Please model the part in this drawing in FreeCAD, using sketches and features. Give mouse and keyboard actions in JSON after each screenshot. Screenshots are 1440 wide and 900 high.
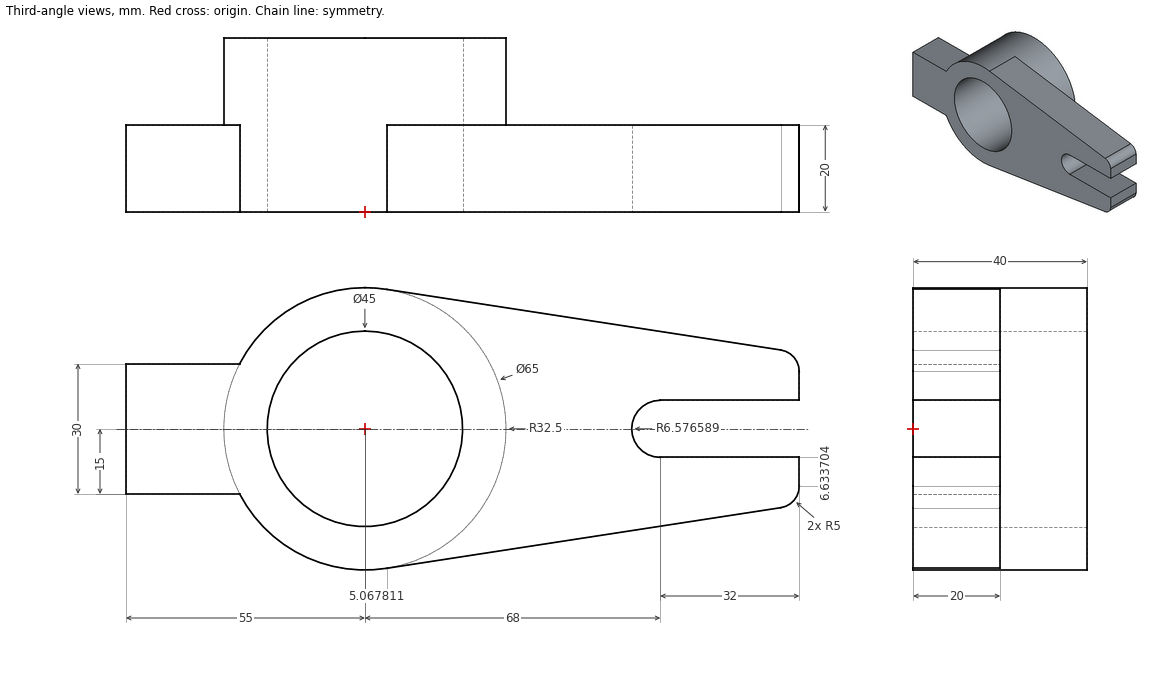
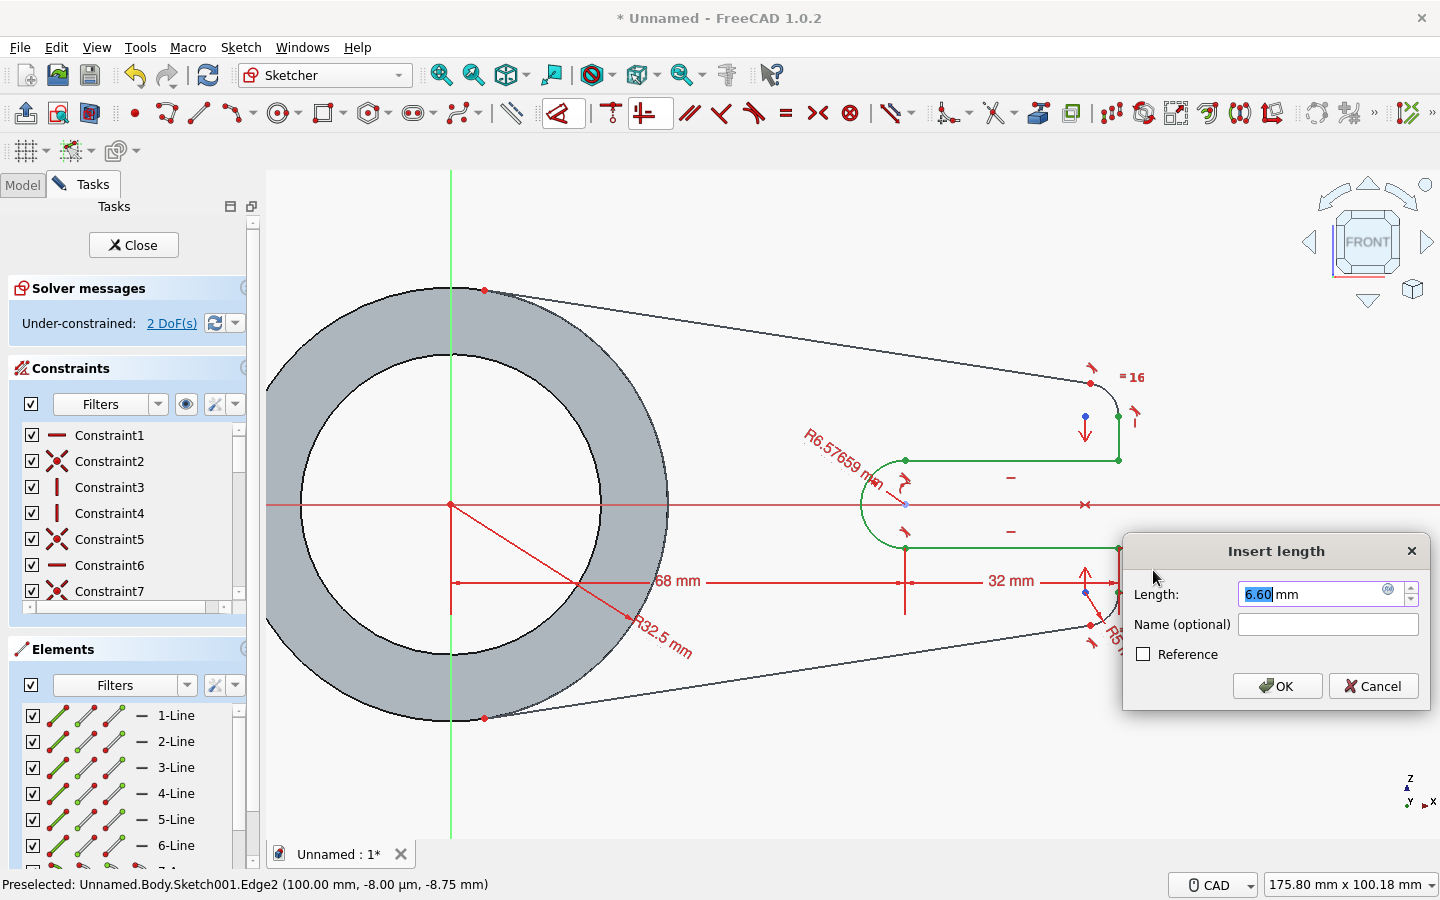
{"action": "type", "text": "6.633704"}
{"action": "key", "text": "Return"}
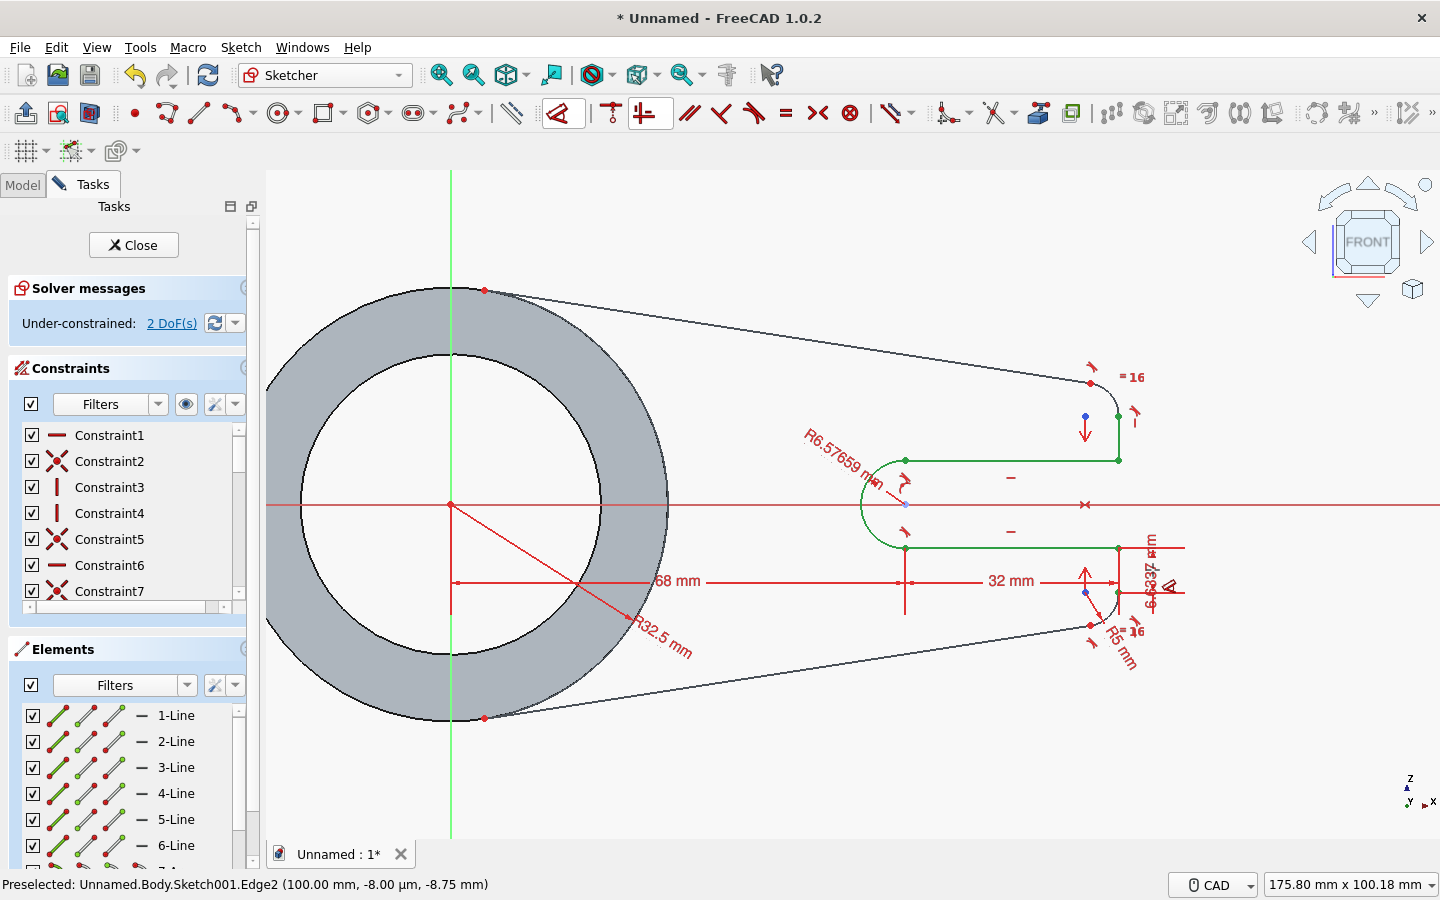
{"action": "left_click", "coordinate": [485, 719]}
{"action": "left_click", "coordinate": [468, 753]}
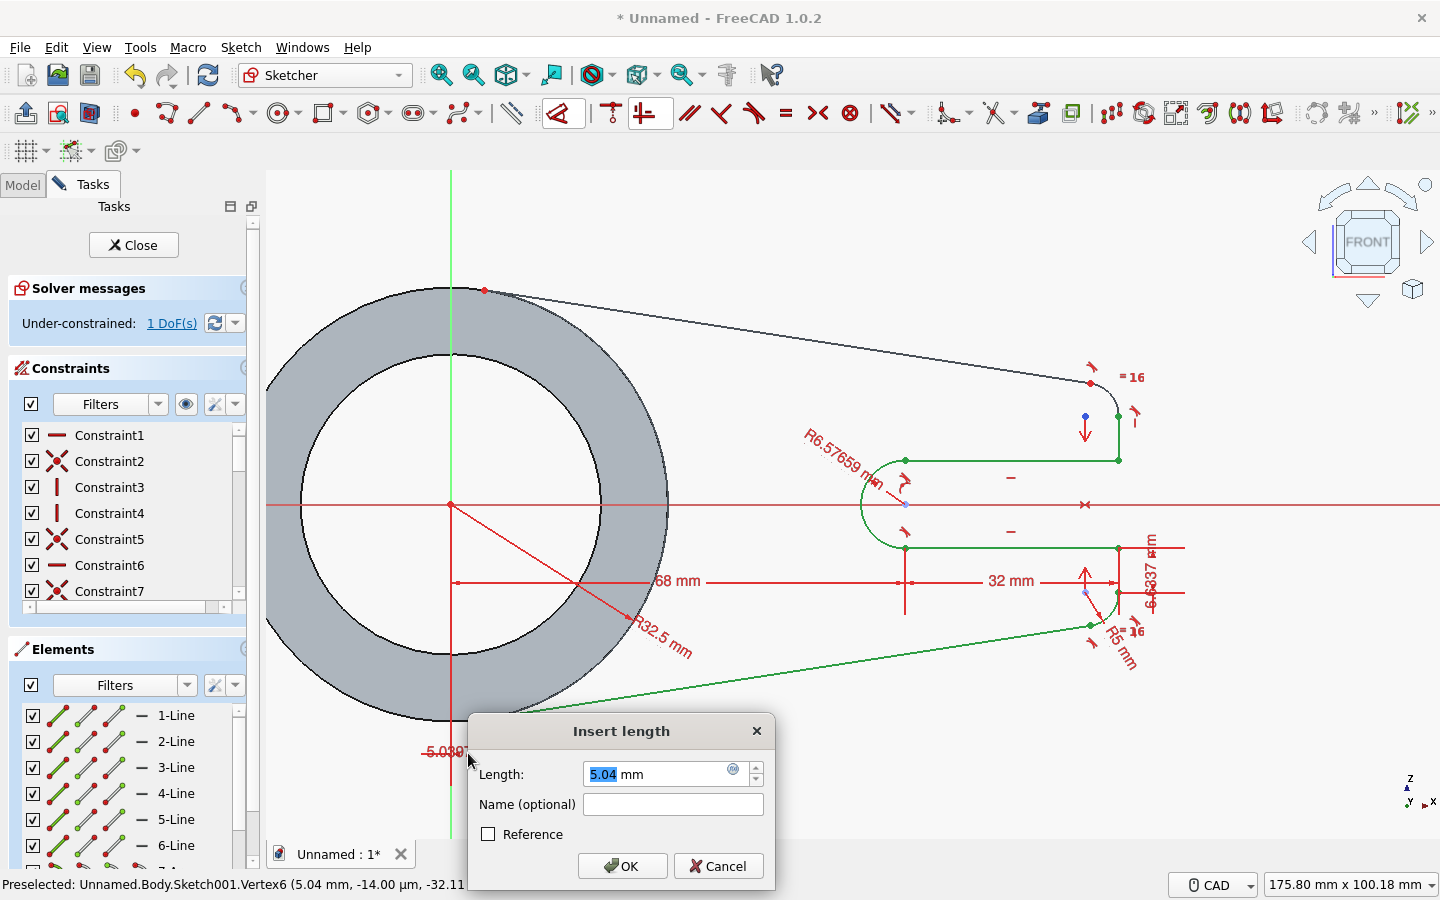
{"action": "type", "text": "5.067811"}
{"action": "key", "text": "Return"}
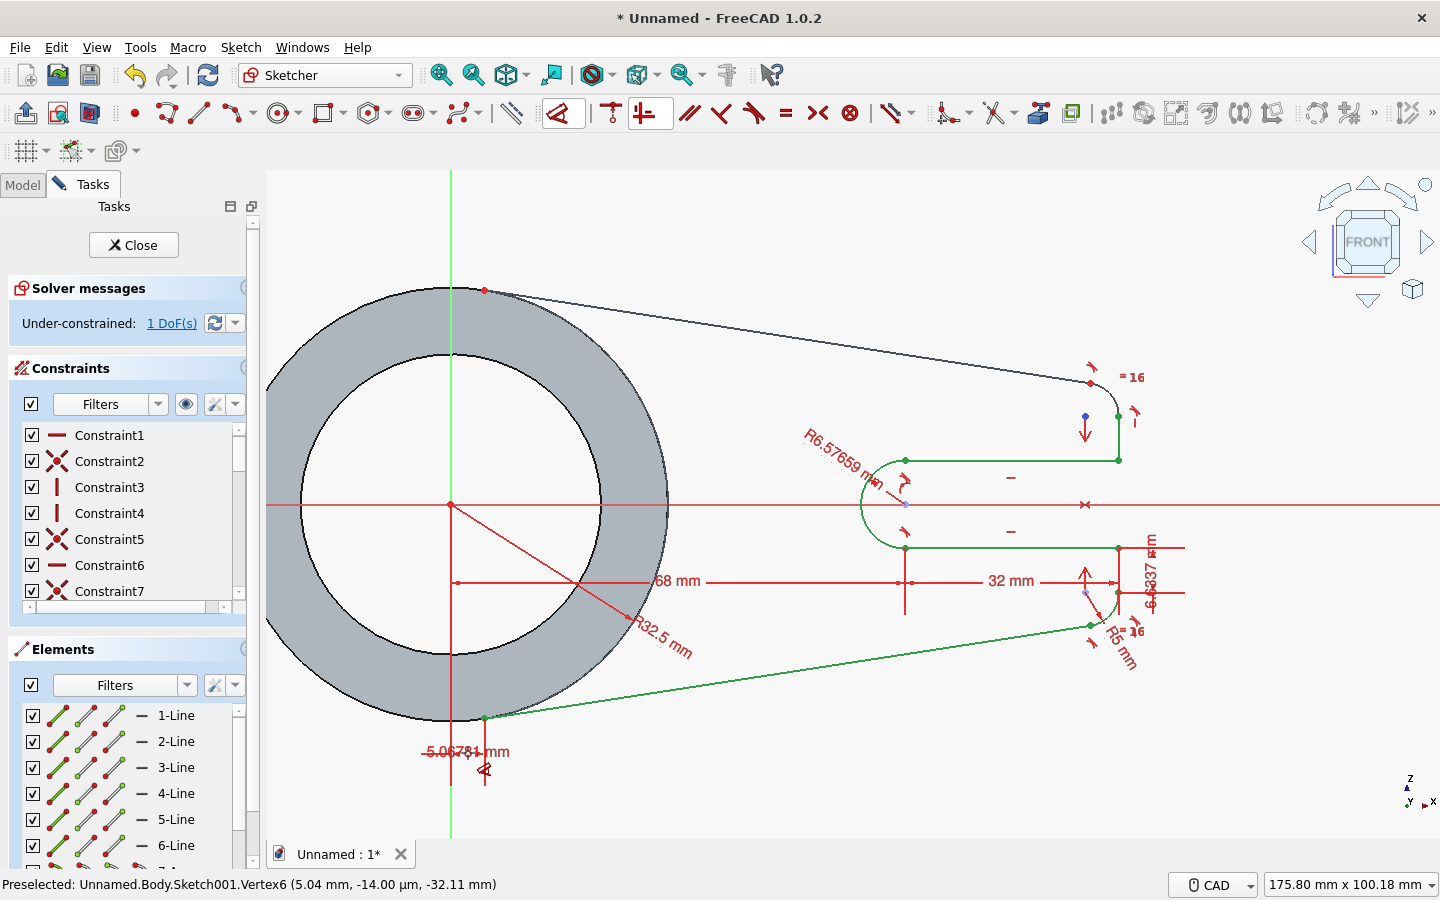
{"action": "left_click", "coordinate": [485, 290]}
{"action": "left_click", "coordinate": [468, 256]}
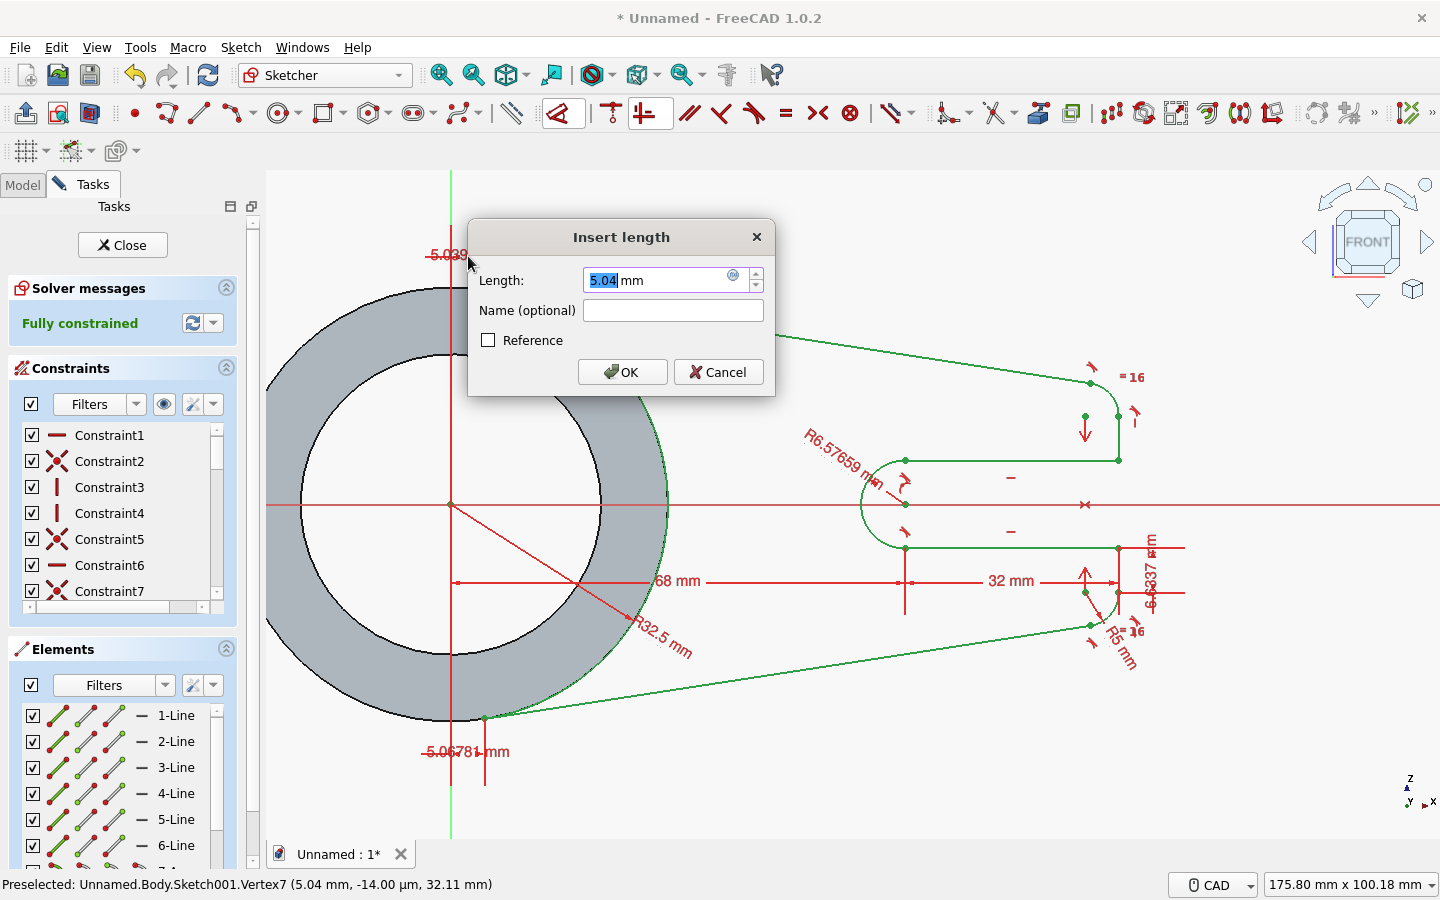
{"action": "type", "text": "5.067811"}
{"action": "key", "text": "Return"}
{"action": "key", "text": "Escape"}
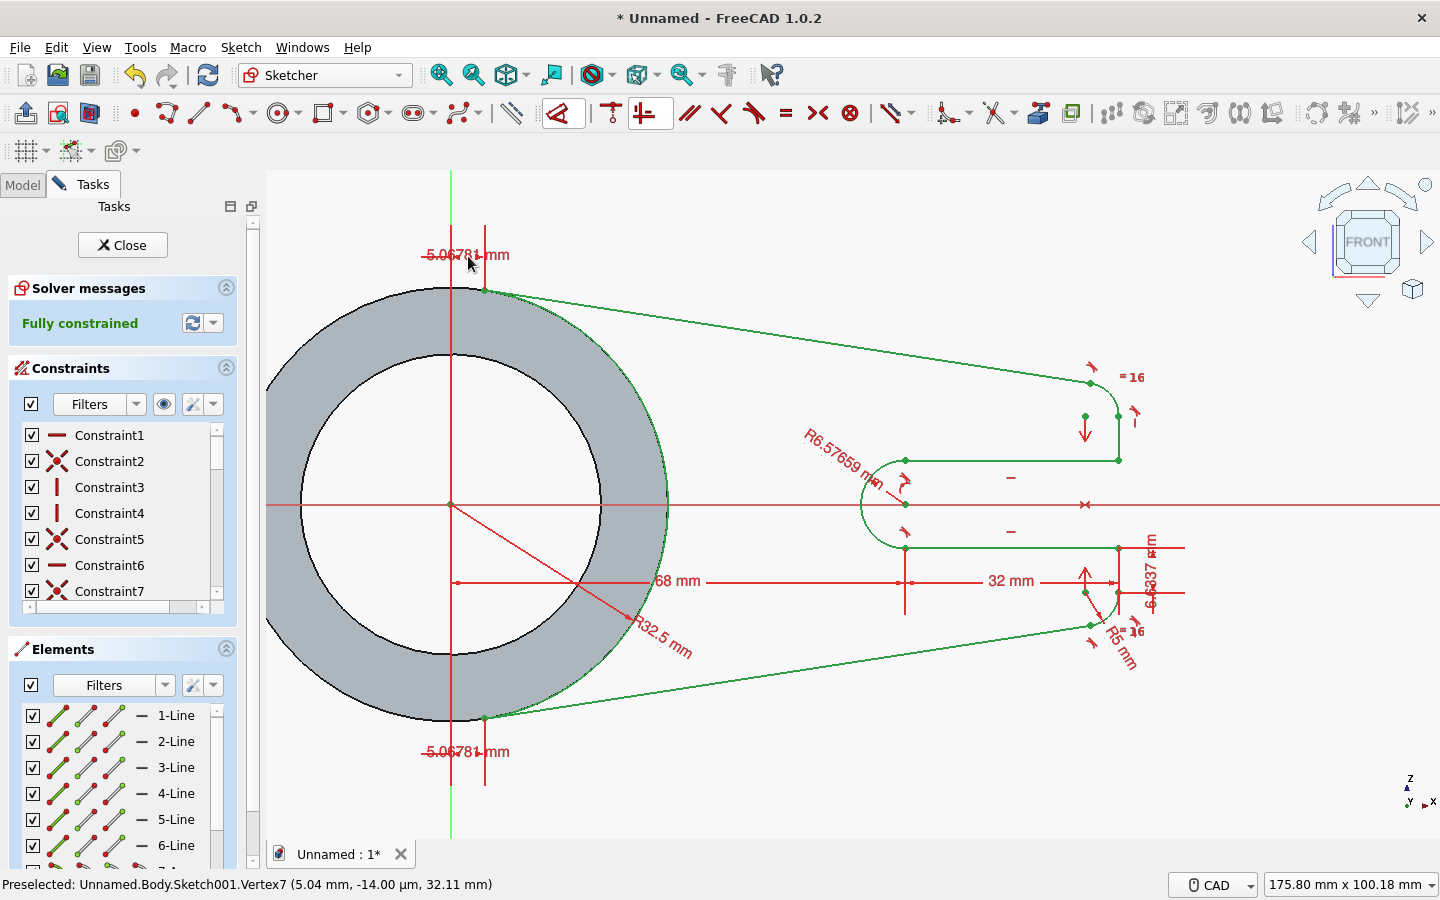
{"action": "left_click", "coordinate": [123, 245]}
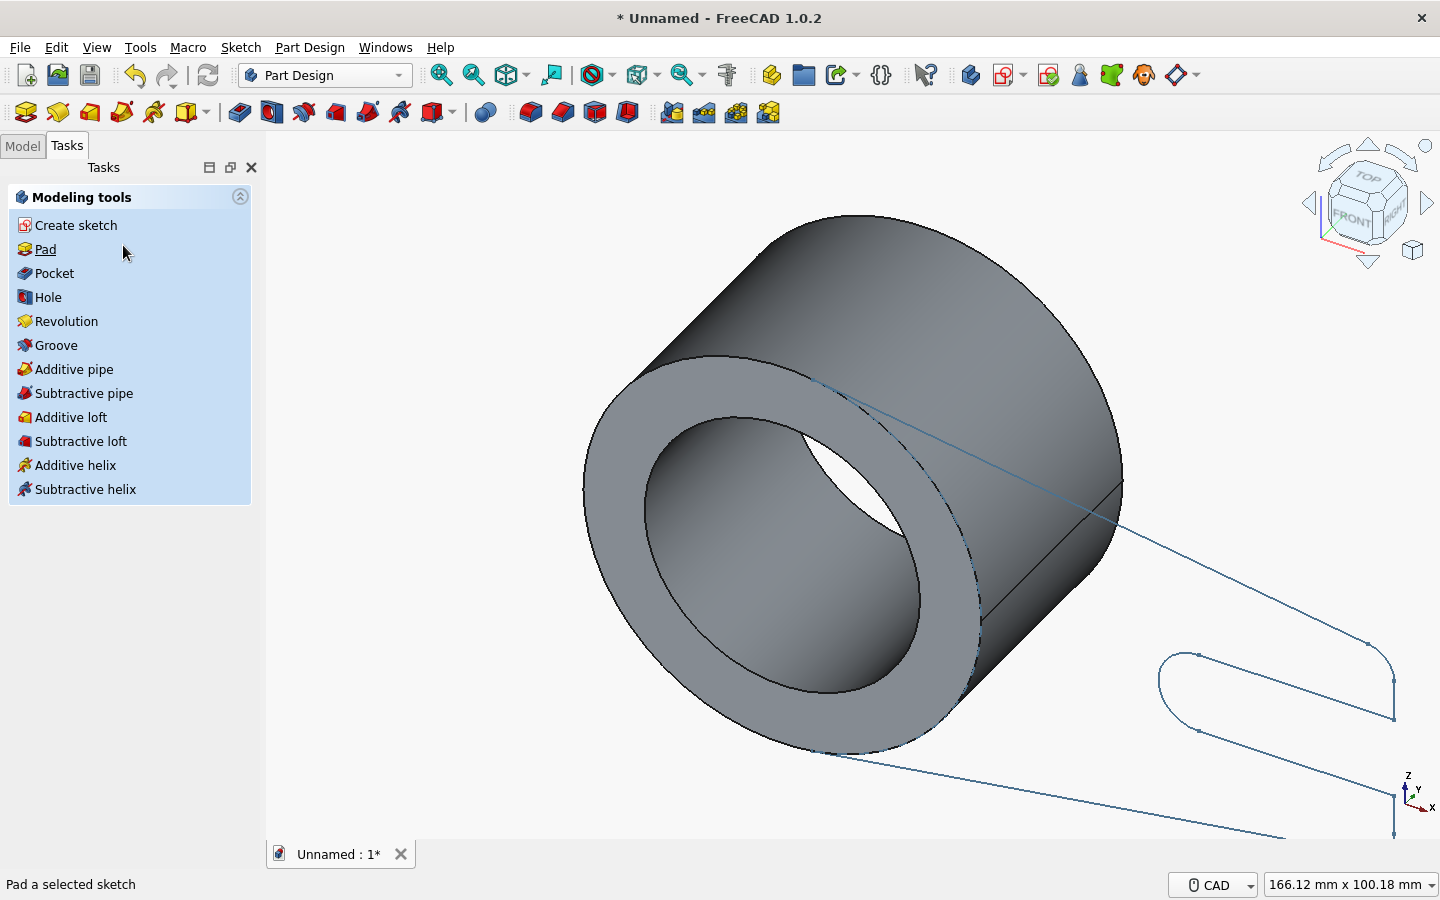
{"action": "left_click", "coordinate": [26, 112]}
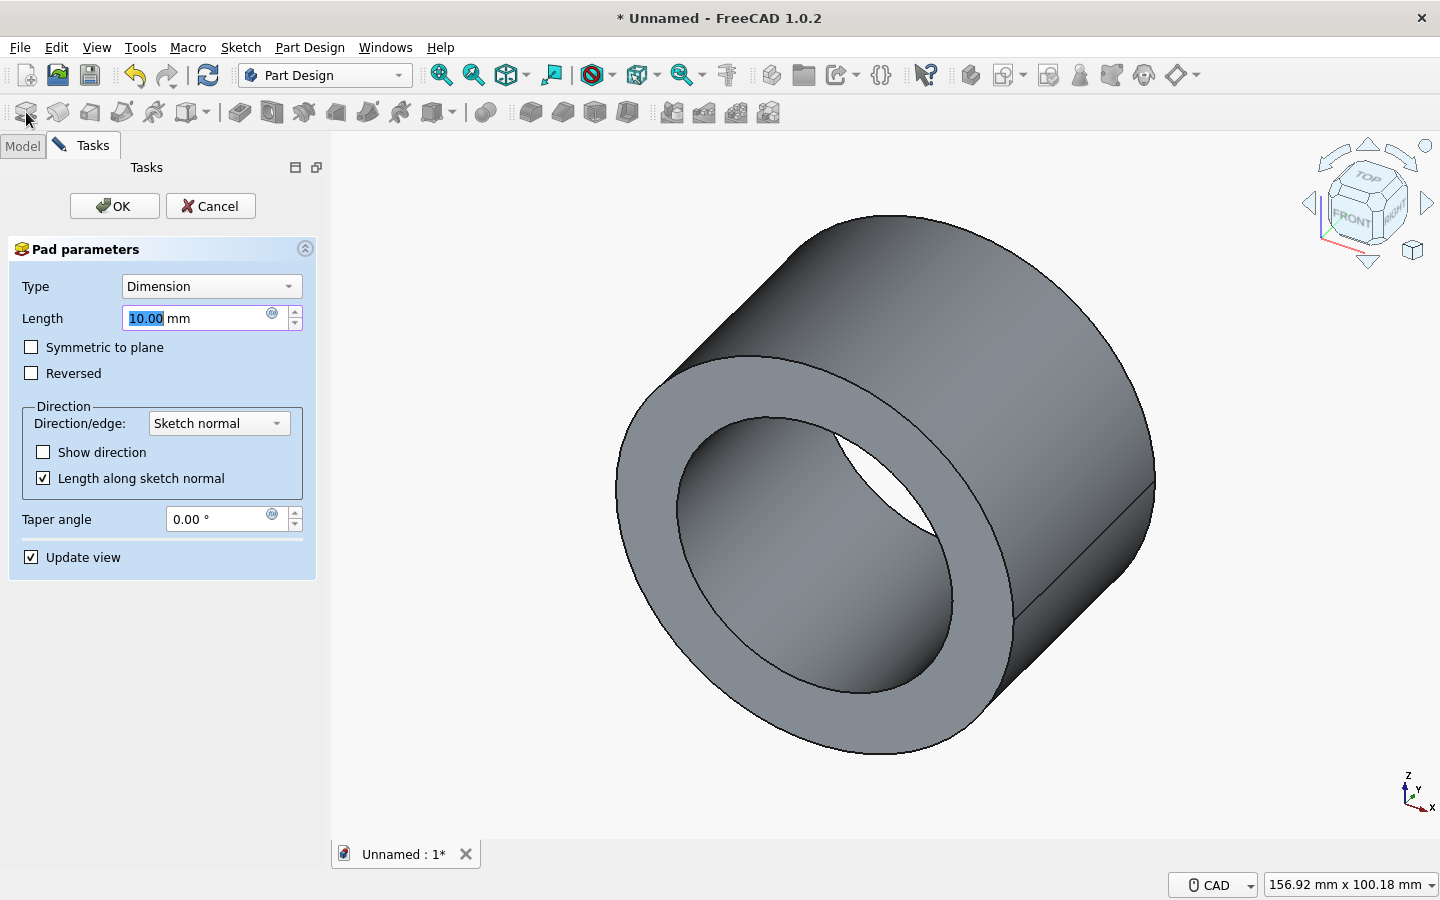
{"action": "type", "text": "20"}
{"action": "key", "text": "Tab"}